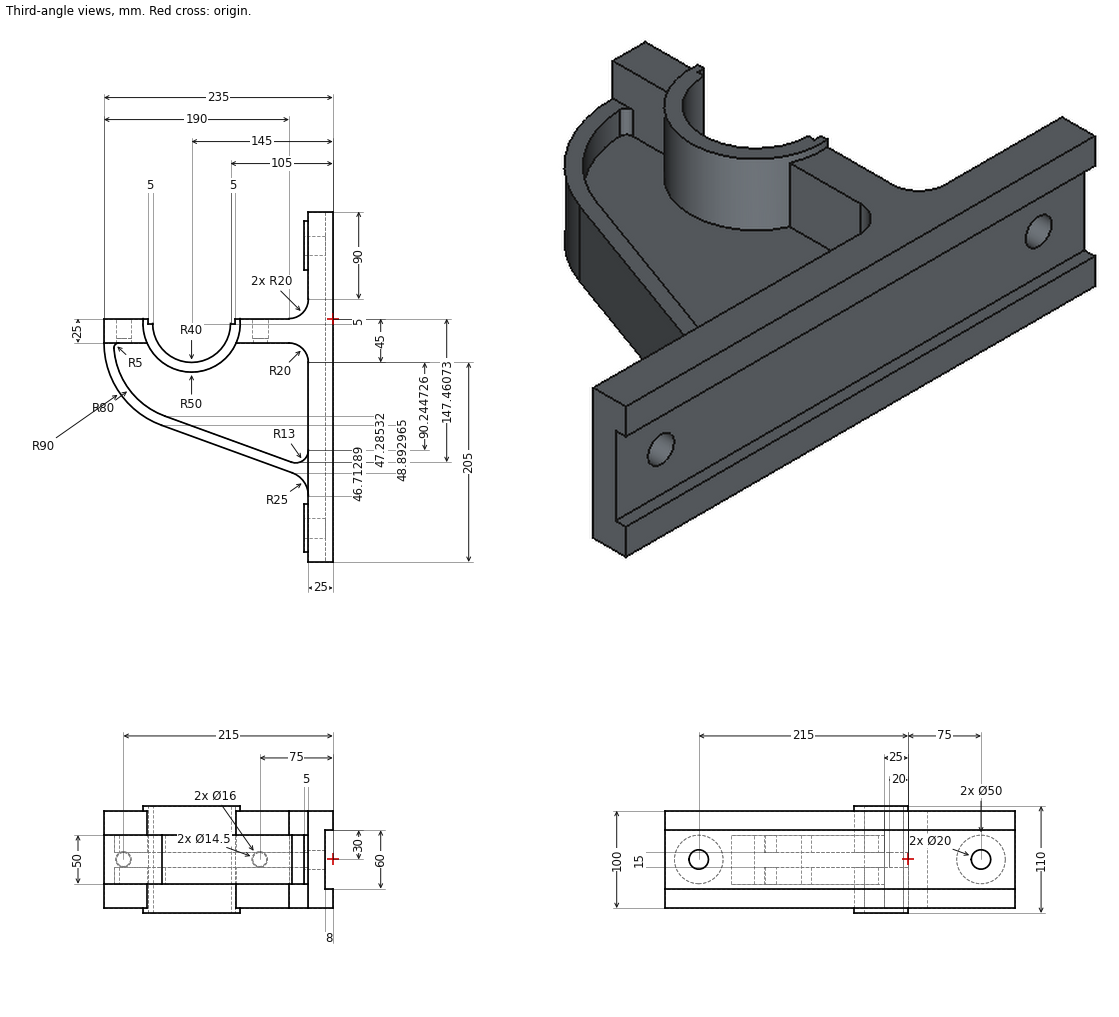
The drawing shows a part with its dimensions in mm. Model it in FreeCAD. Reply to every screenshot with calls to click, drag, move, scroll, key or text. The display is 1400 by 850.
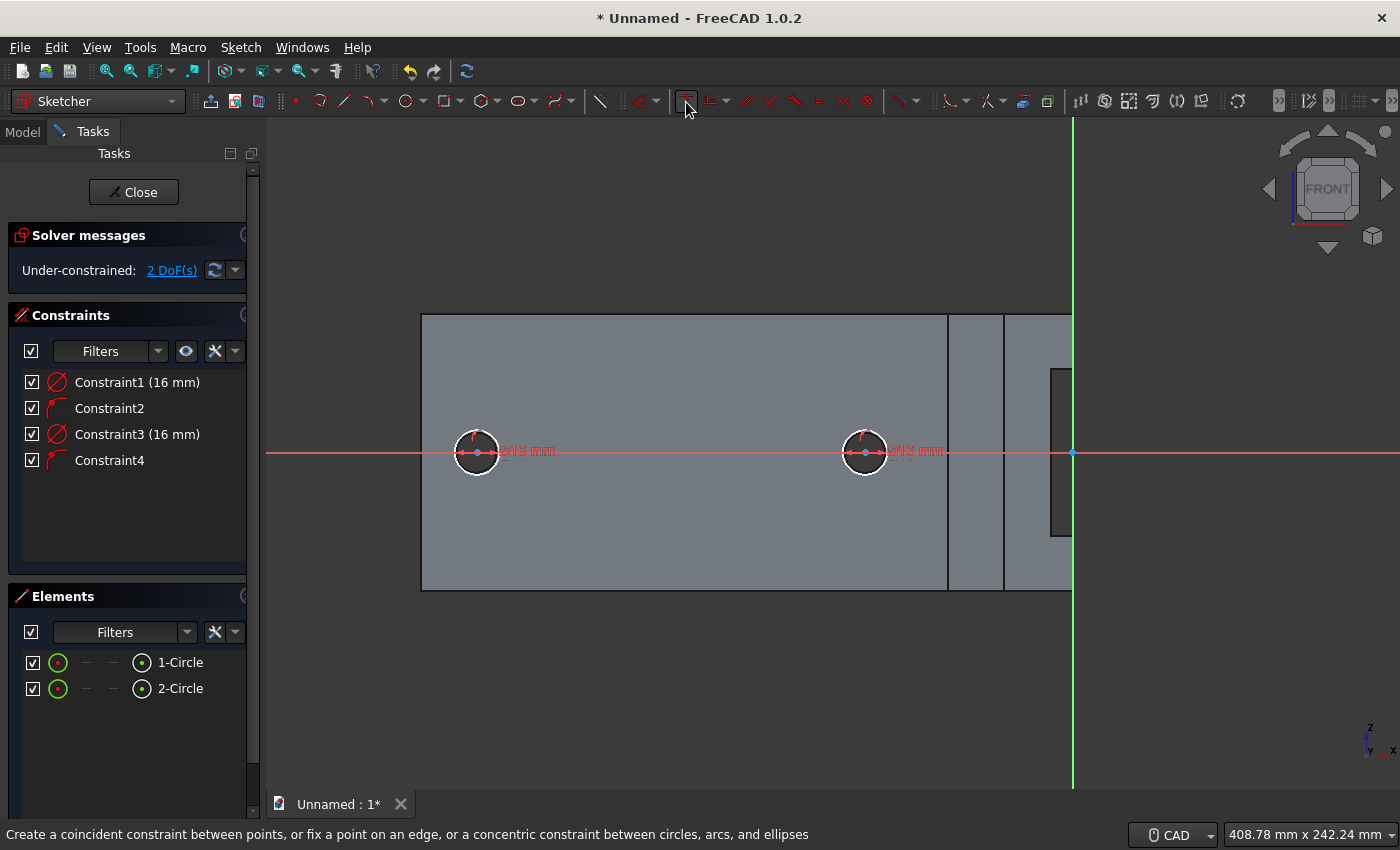
click(640, 102)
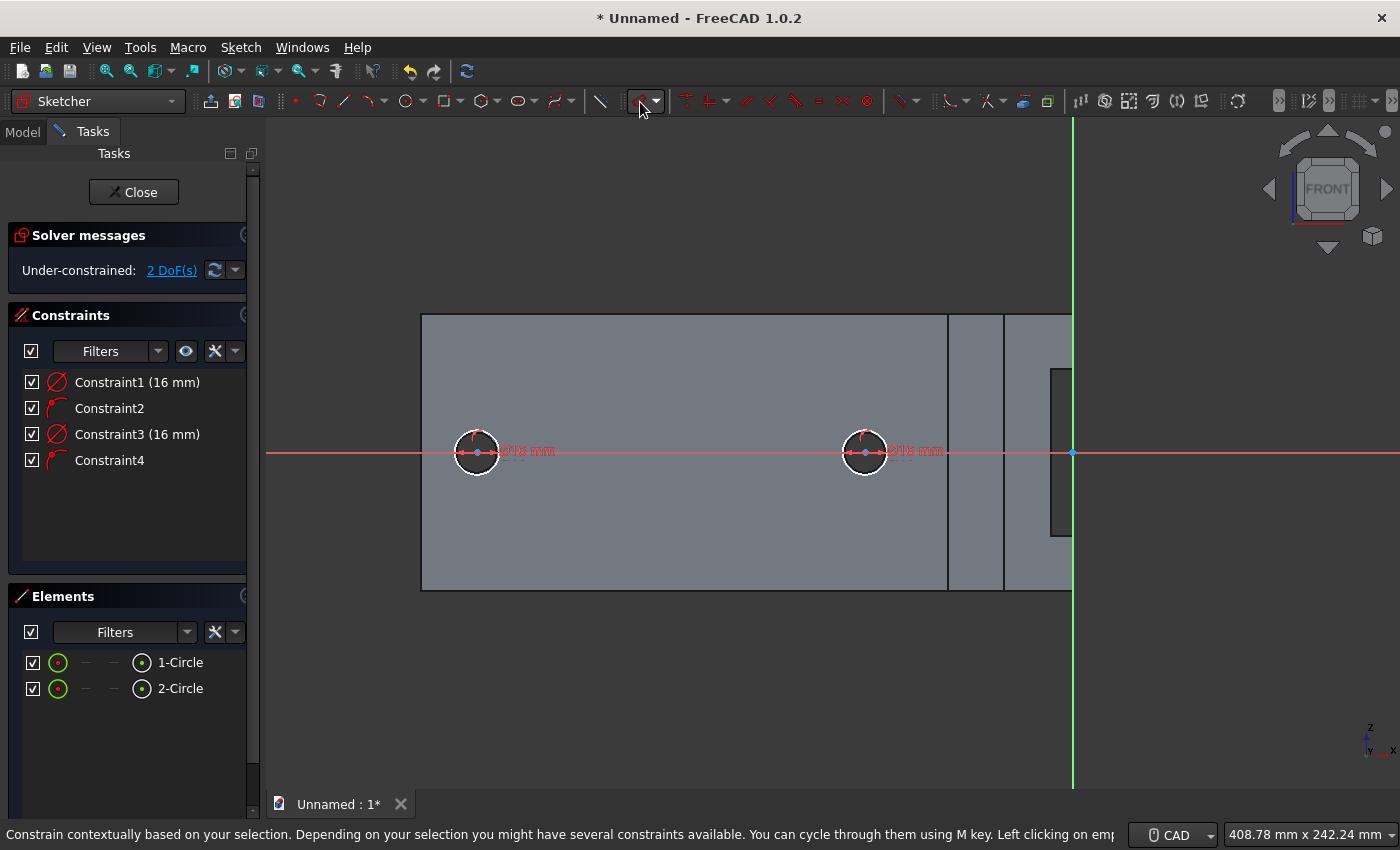
click(865, 453)
click(969, 487)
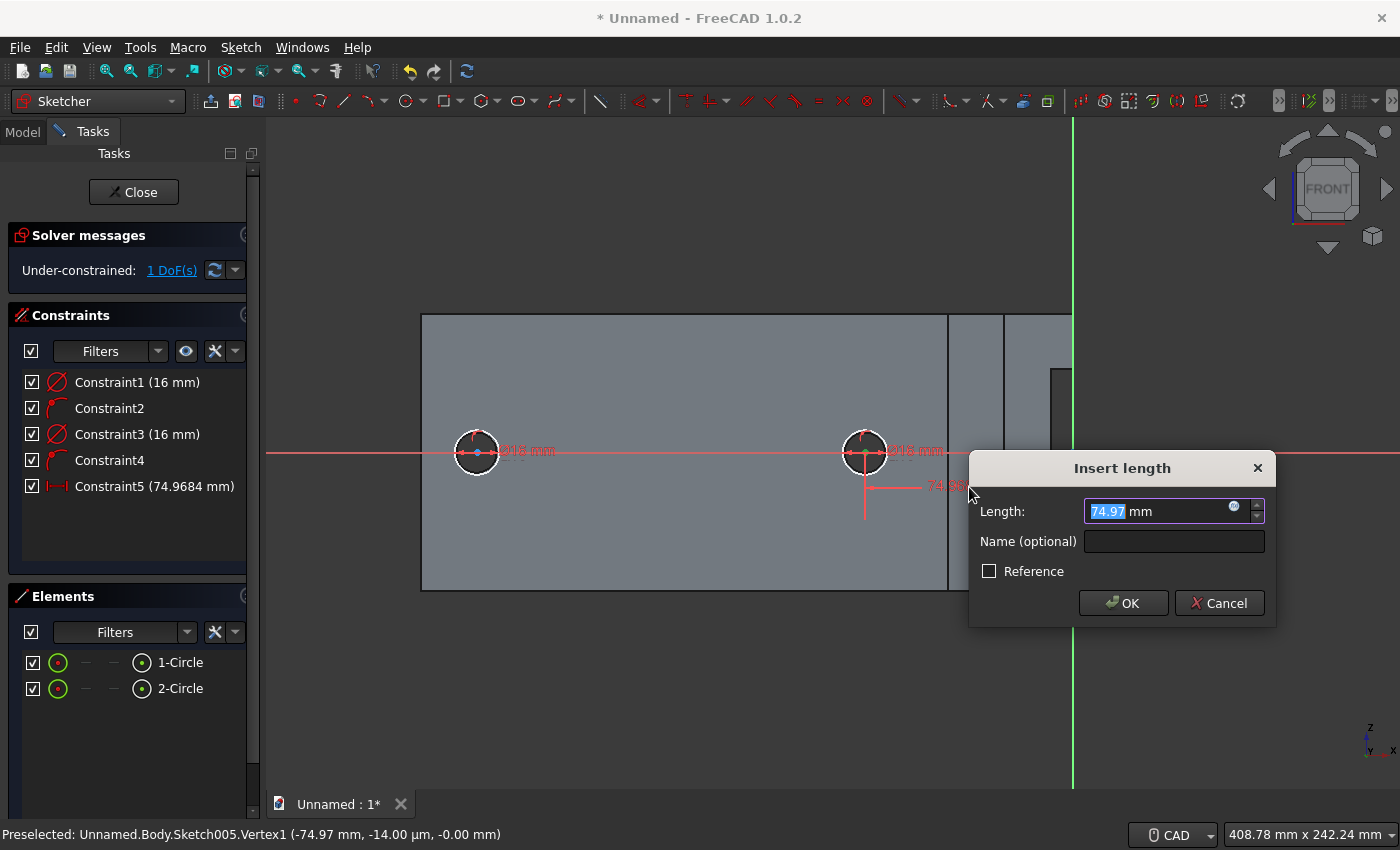
text(75)
key(Return)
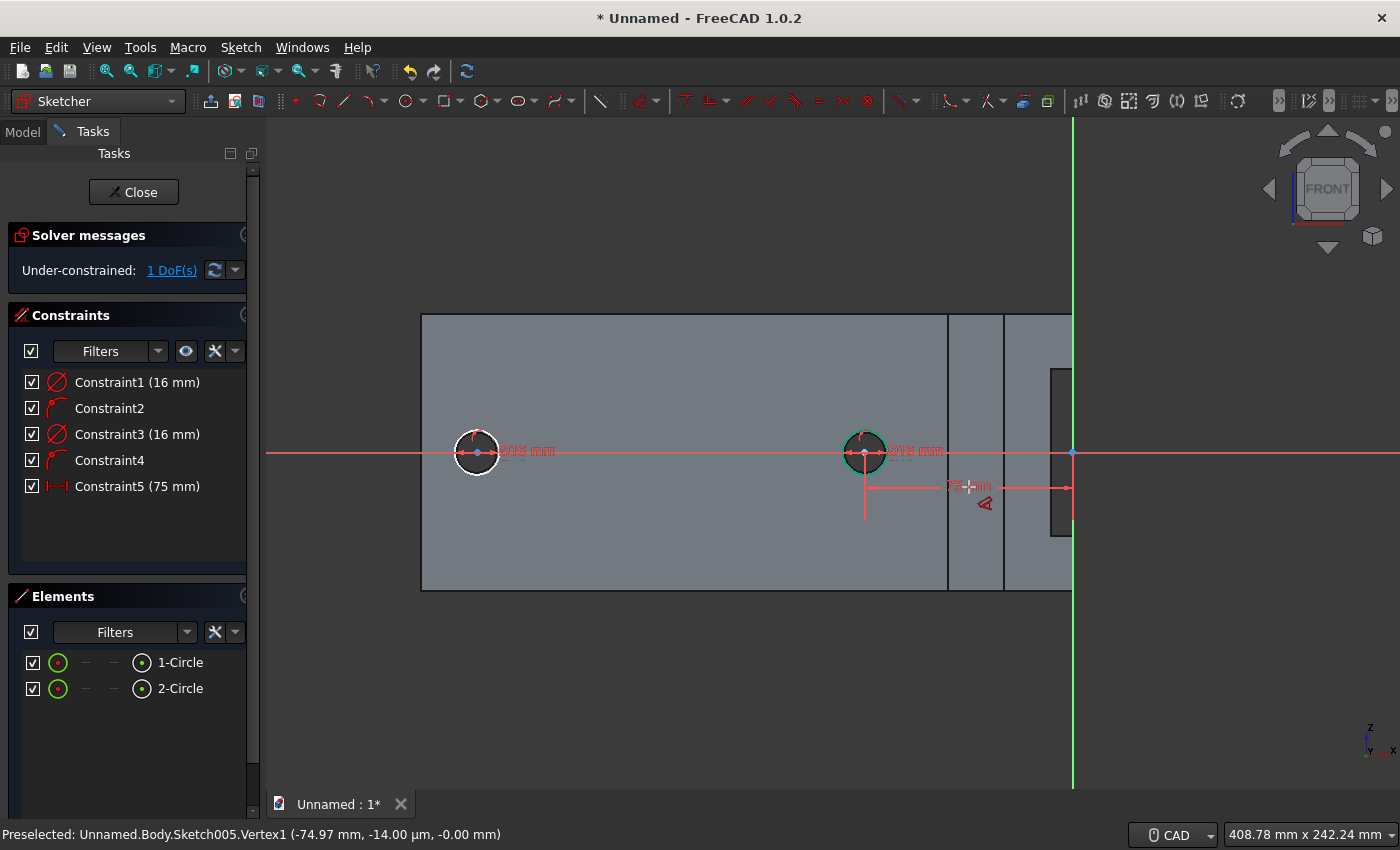
click(477, 453)
click(775, 487)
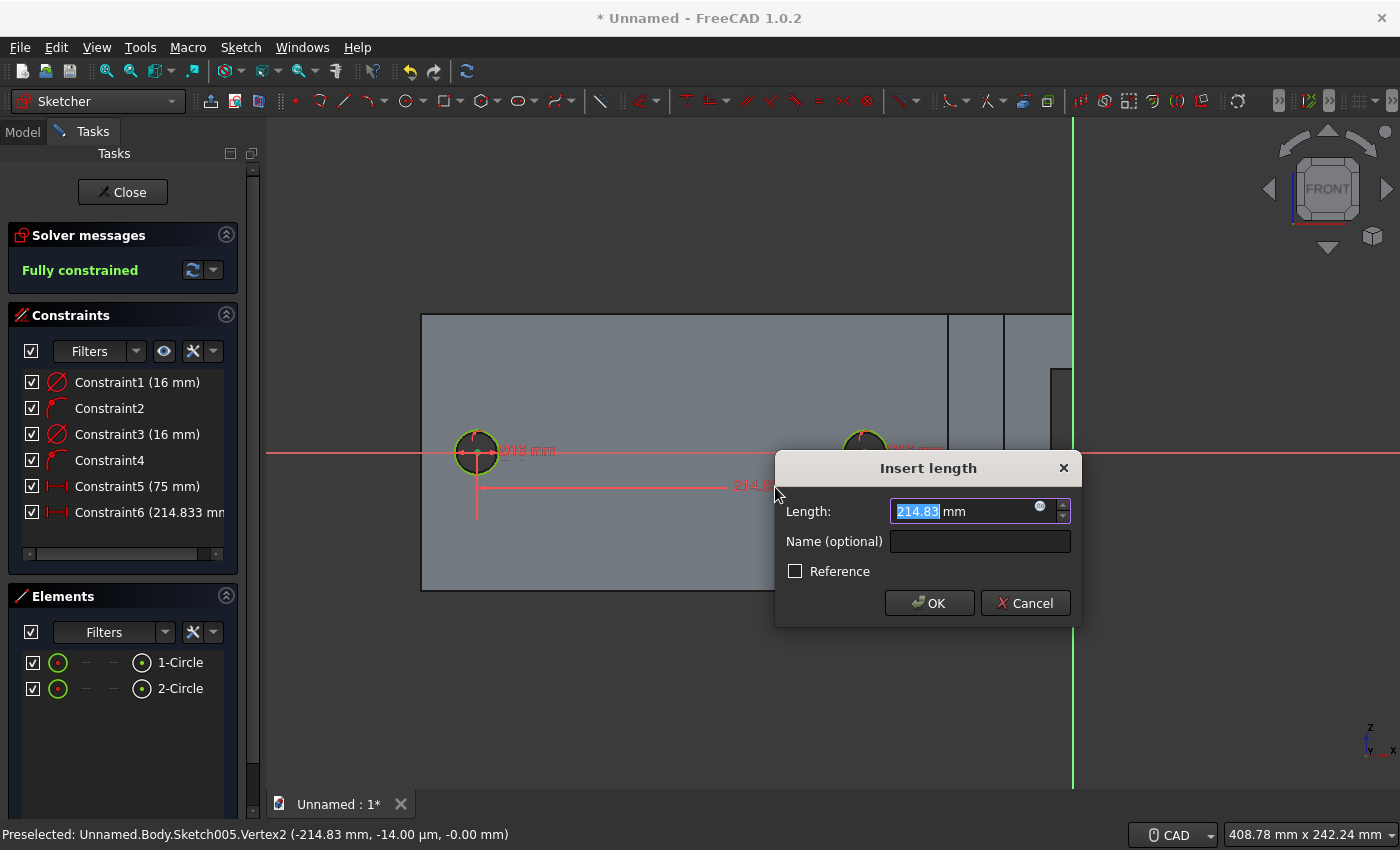
text(215)
key(Return)
key(Escape)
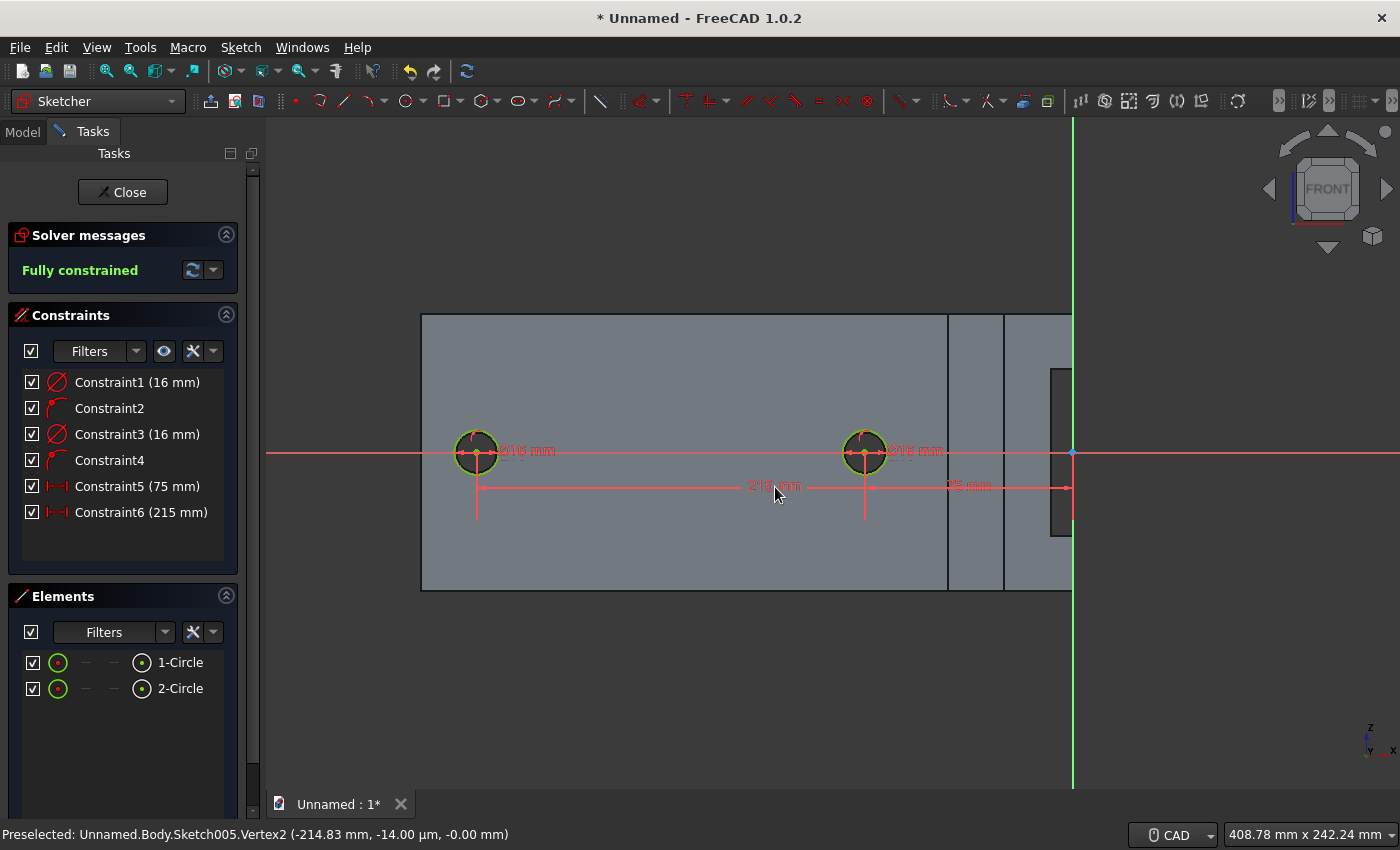
click(123, 192)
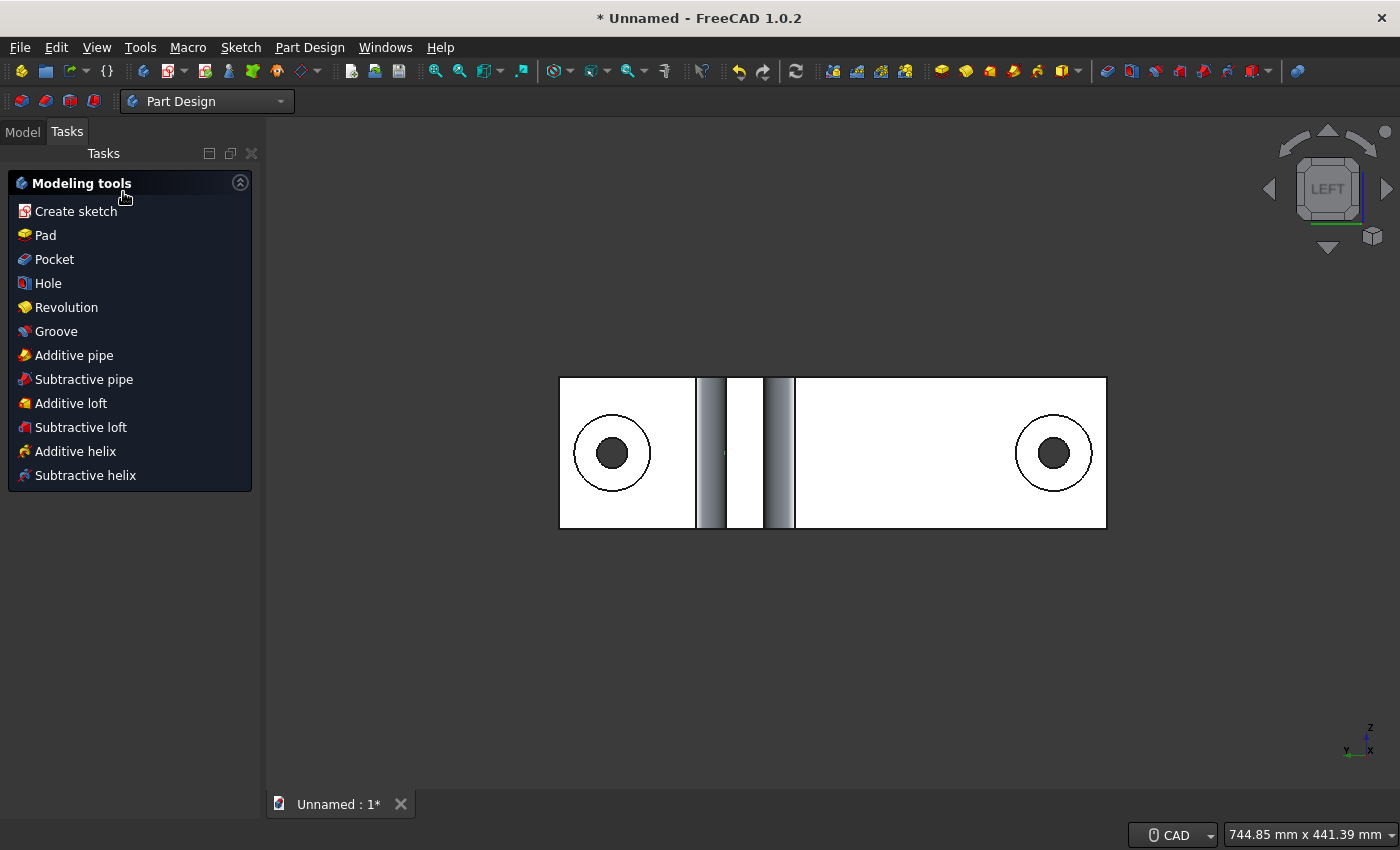
click(1108, 72)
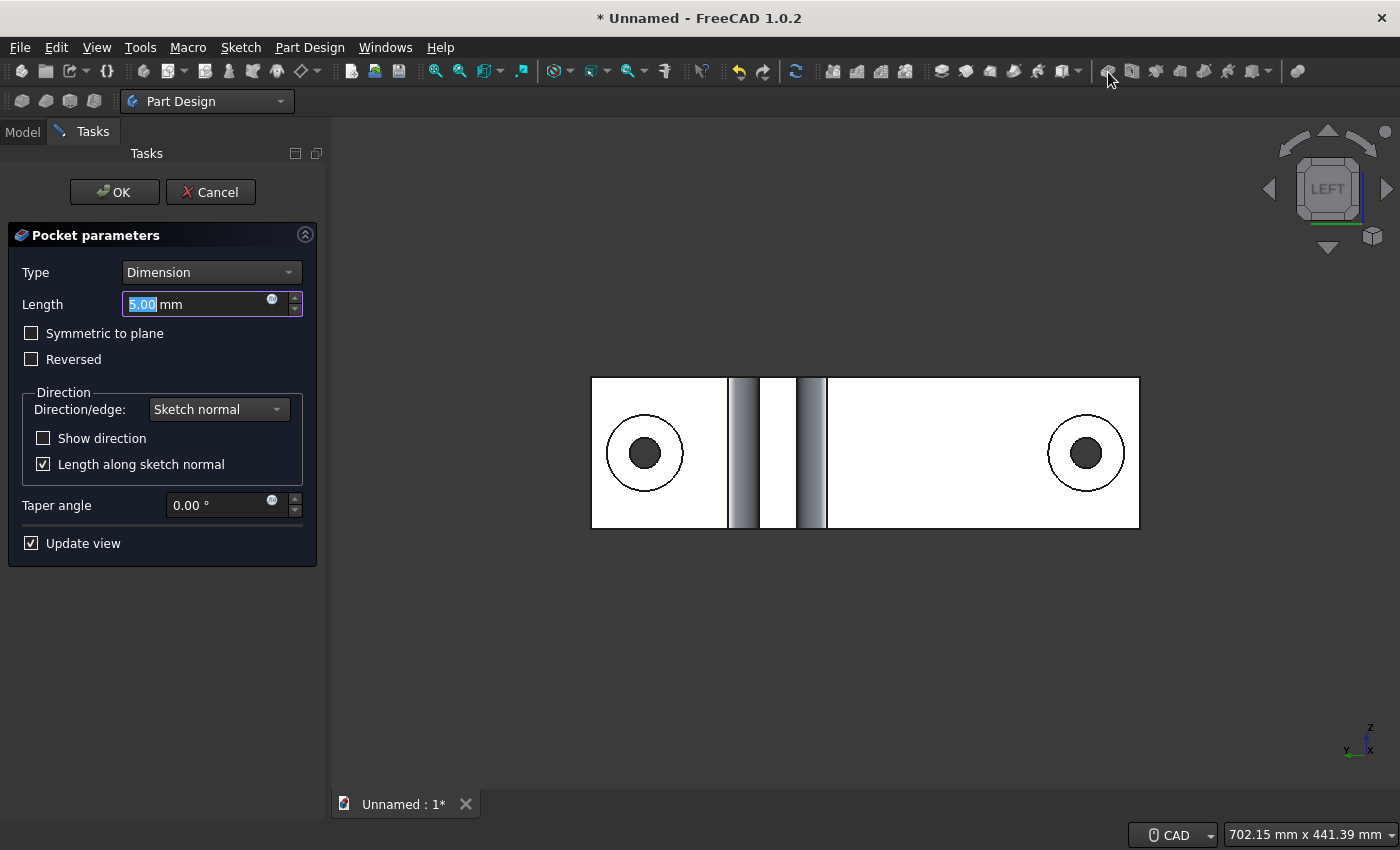
text(20)
key(Tab)